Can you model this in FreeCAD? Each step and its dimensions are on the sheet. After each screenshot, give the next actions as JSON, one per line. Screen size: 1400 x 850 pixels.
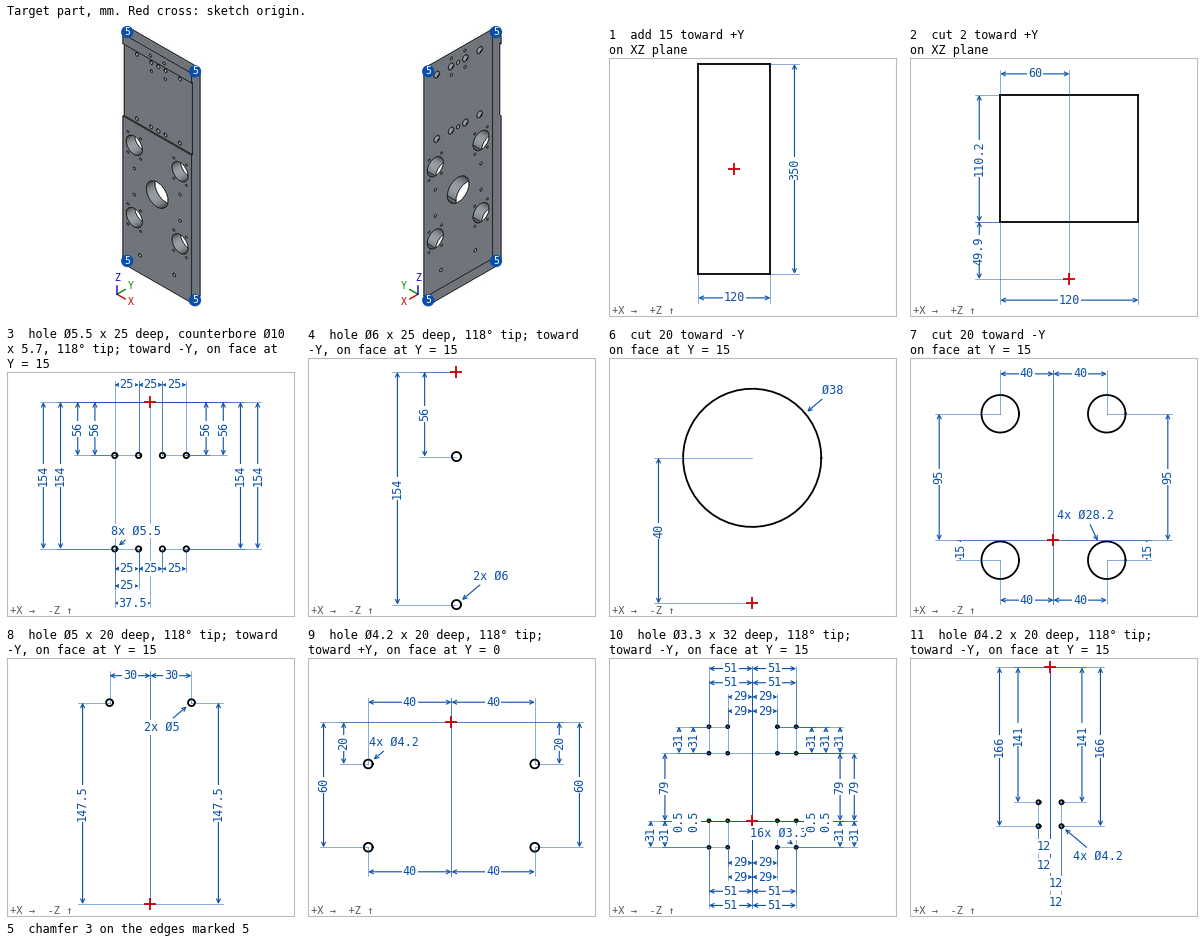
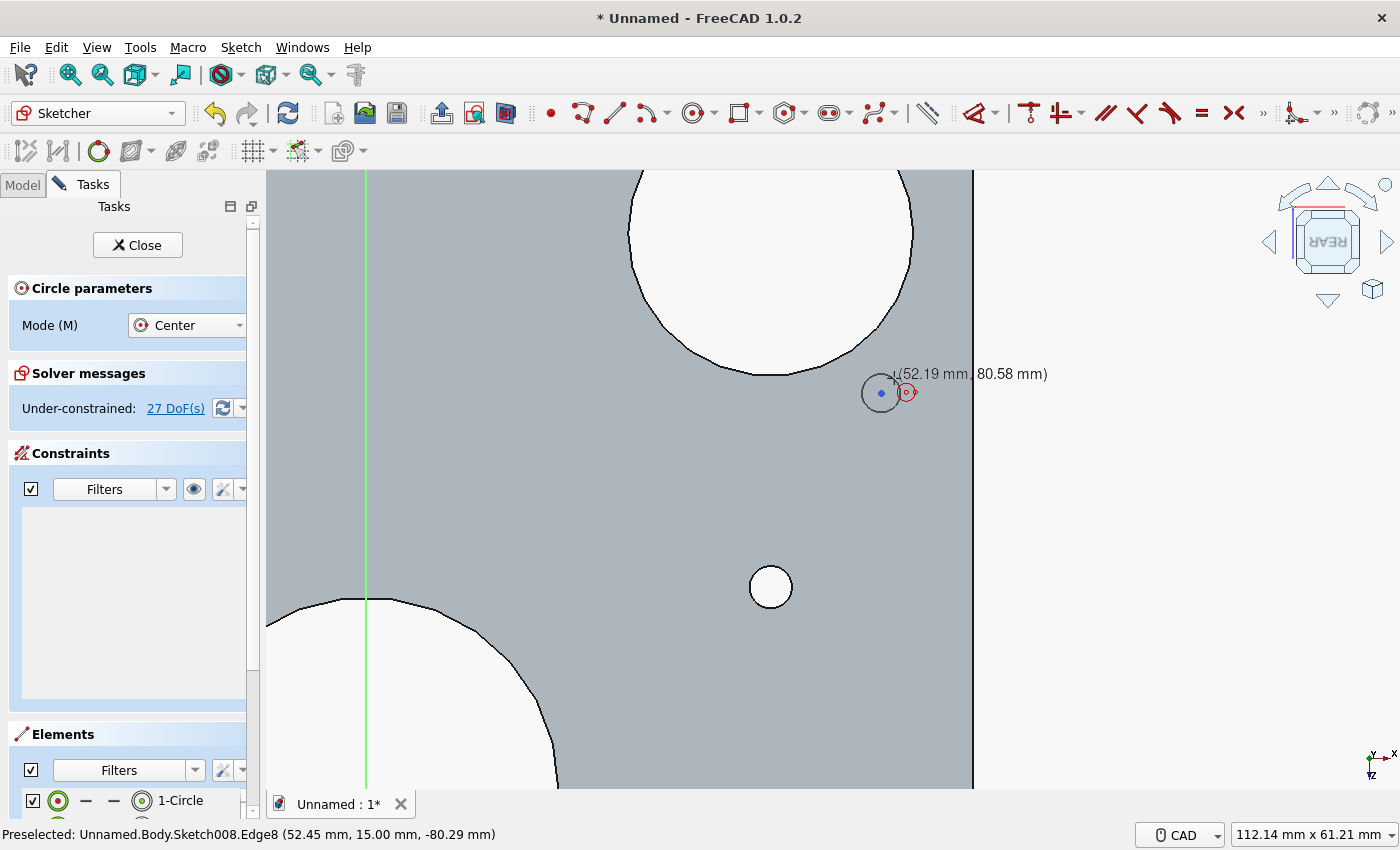
{"action": "scroll", "coordinate": [660, 390], "scroll_direction": "up", "scroll_amount": 2}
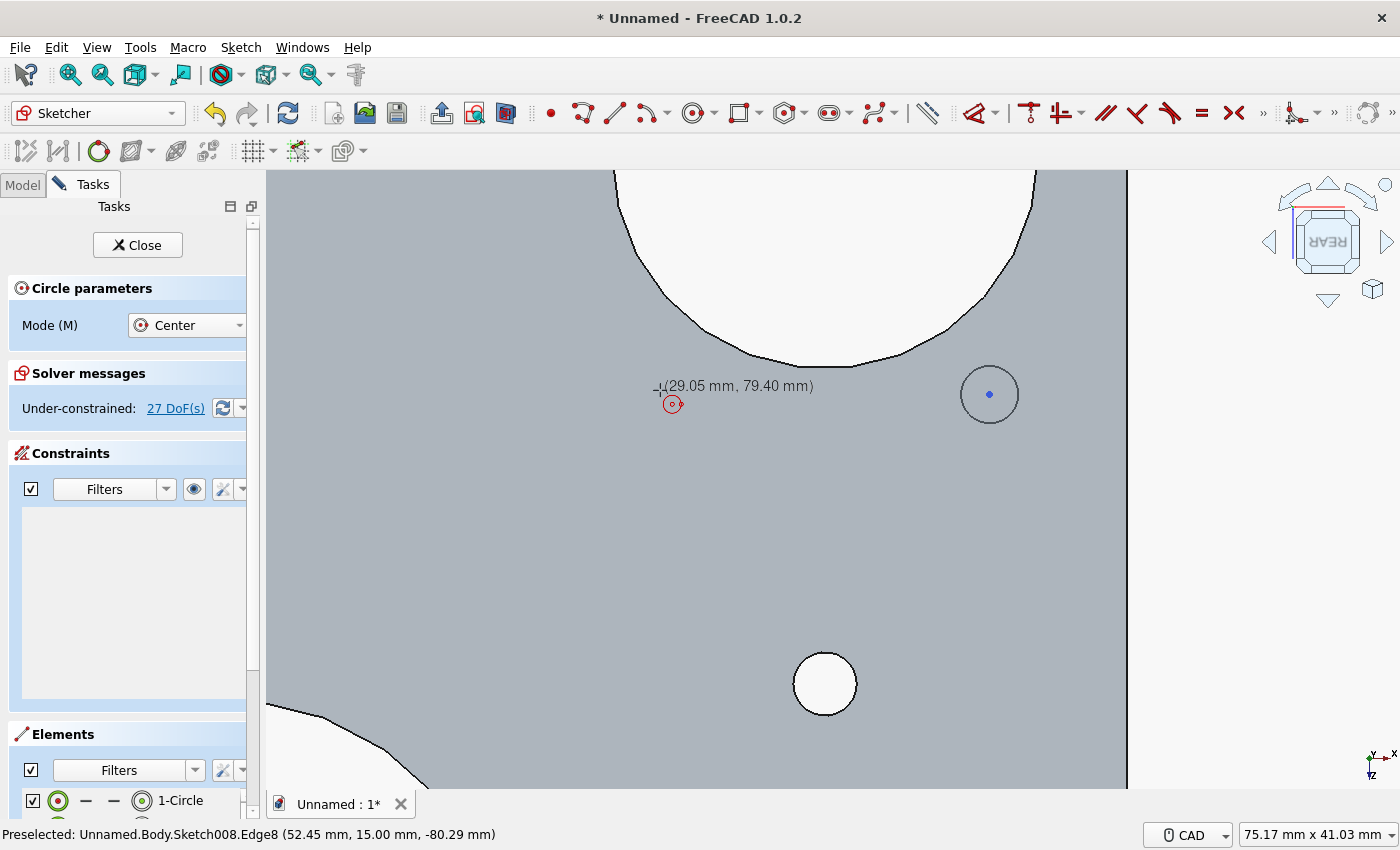
{"action": "scroll", "coordinate": [872, 379], "scroll_direction": "down", "scroll_amount": 9}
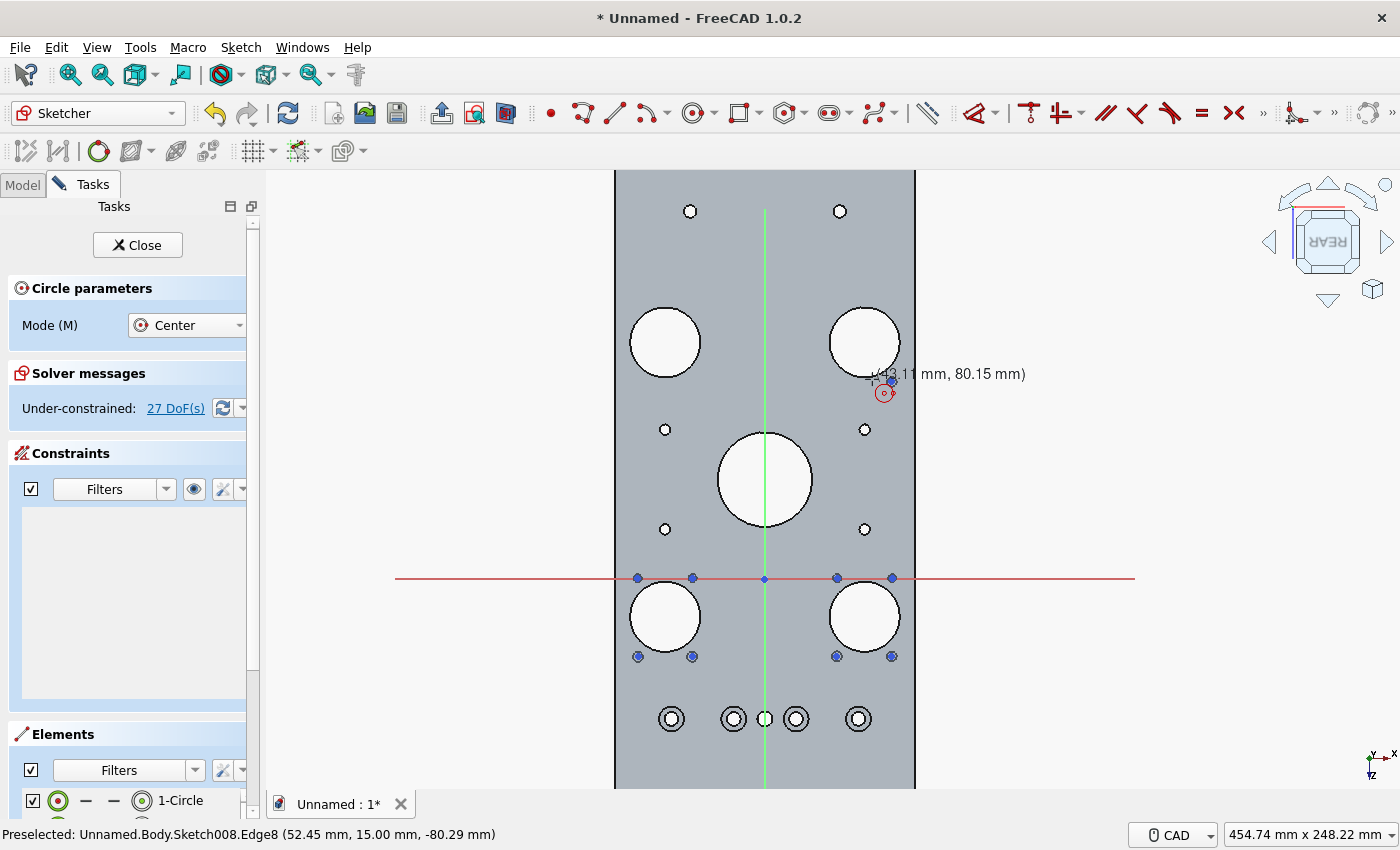
{"action": "left_click", "coordinate": [837, 381]}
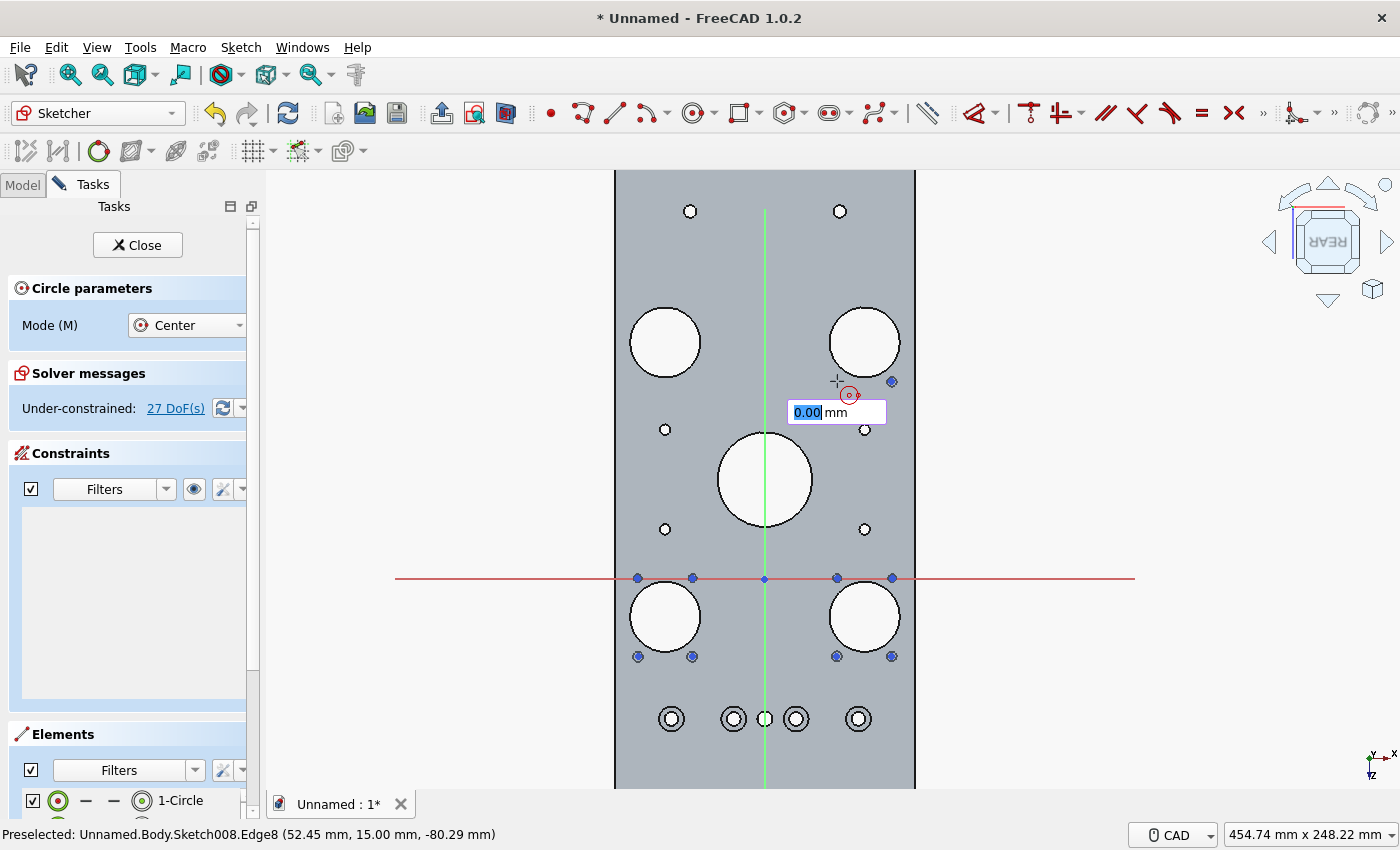
{"action": "scroll", "coordinate": [840, 378], "scroll_direction": "up", "scroll_amount": 7}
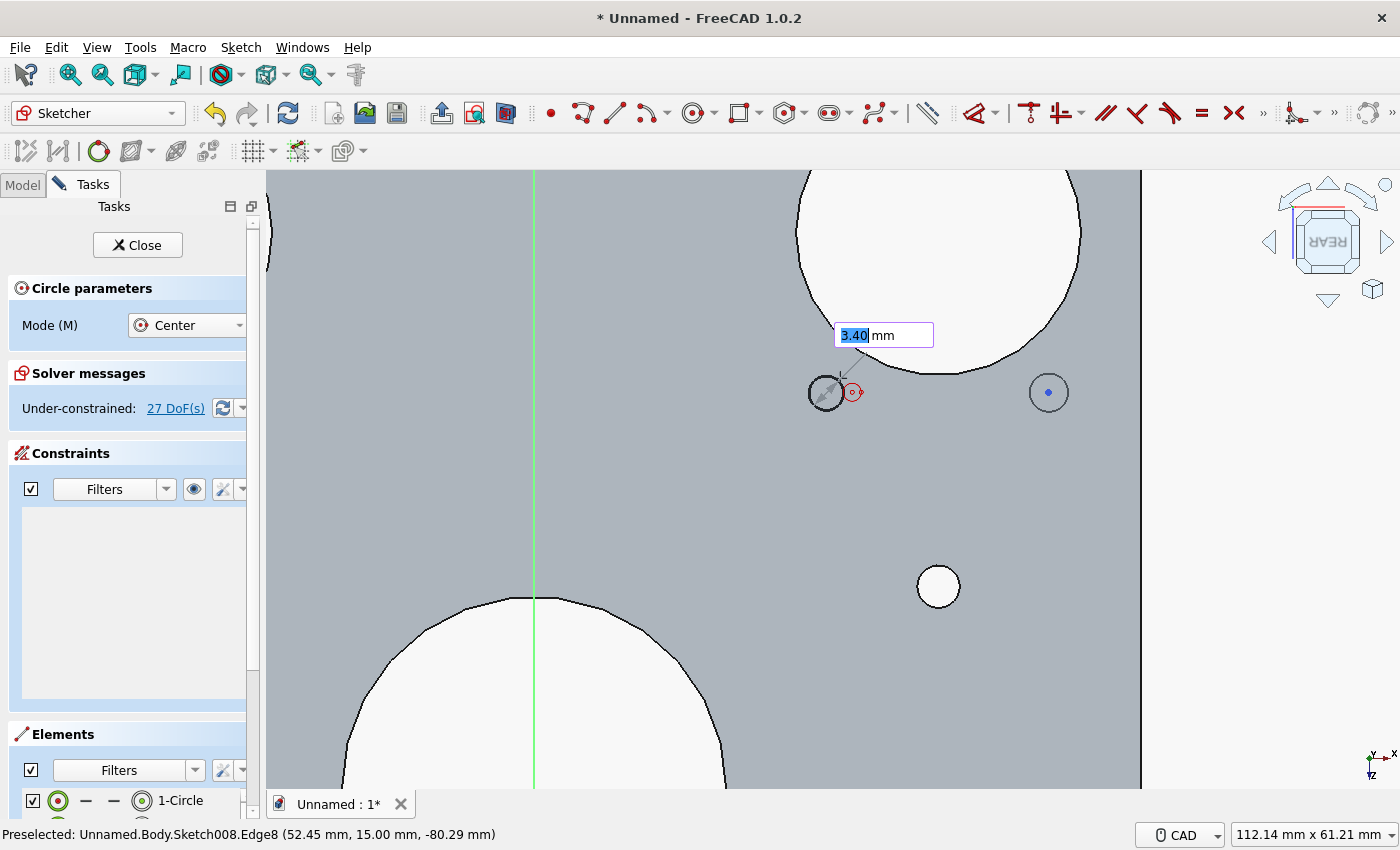
{"action": "left_click", "coordinate": [839, 378]}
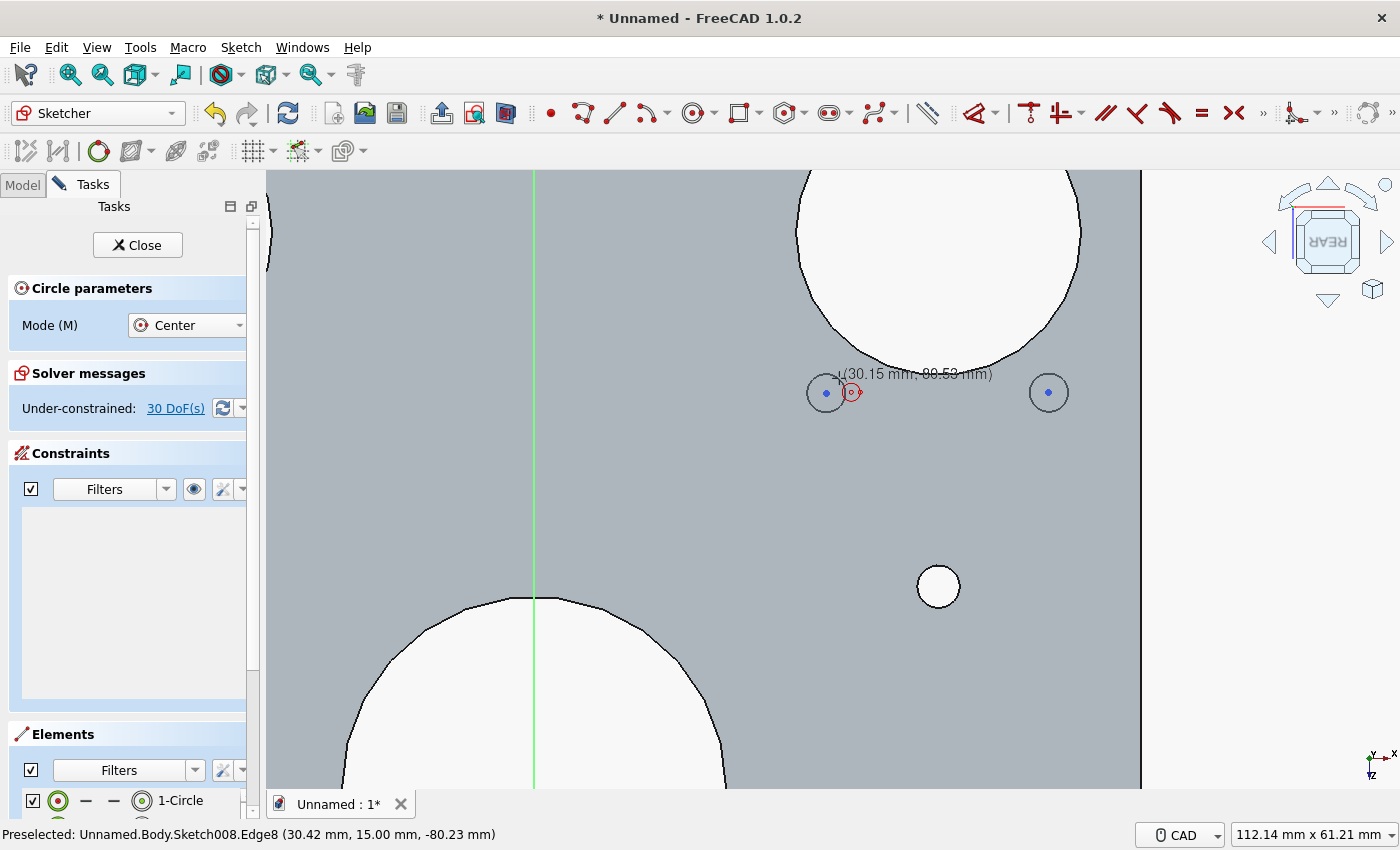
{"action": "scroll", "coordinate": [840, 378], "scroll_direction": "down", "scroll_amount": 7}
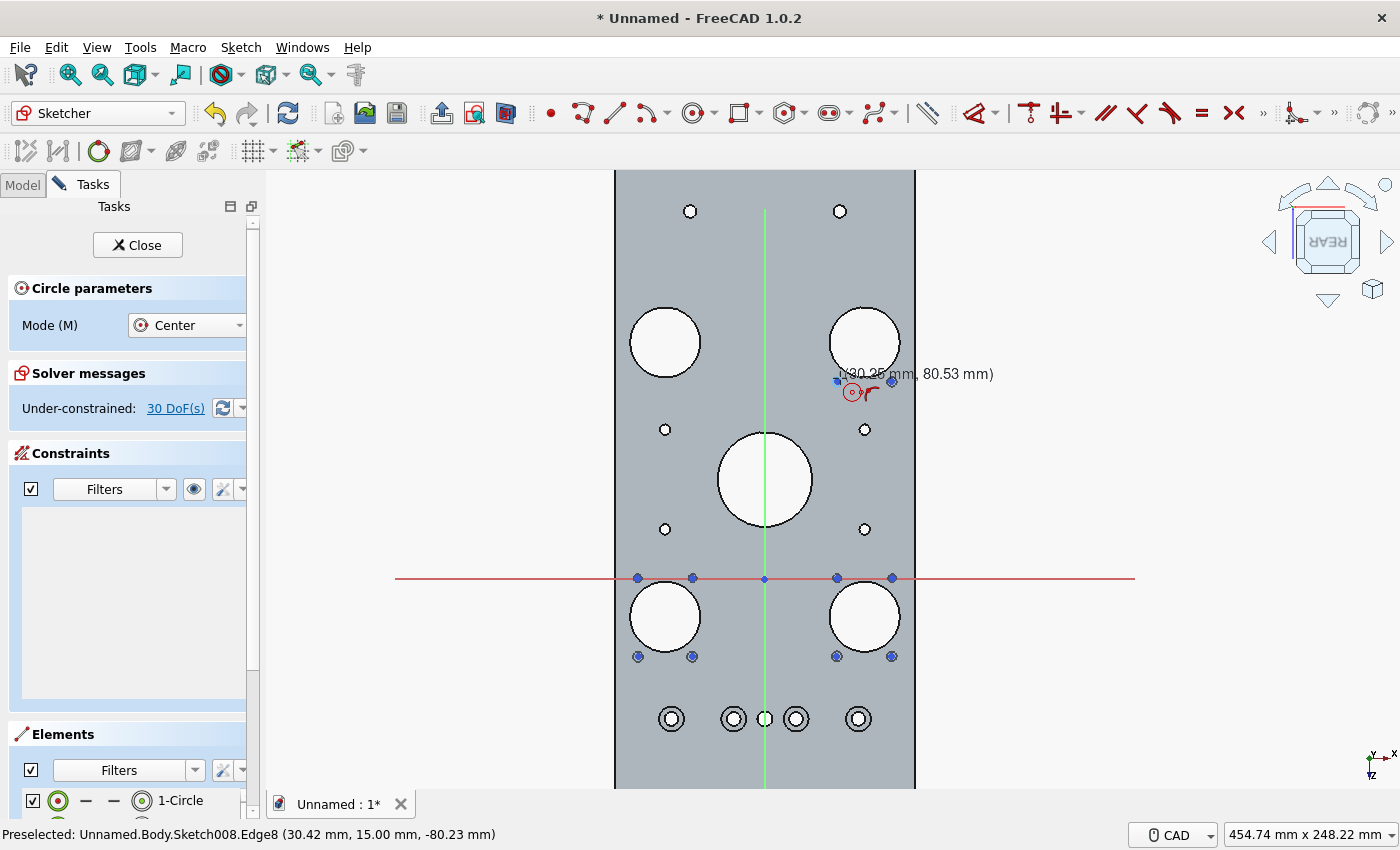
{"action": "scroll", "coordinate": [892, 304], "scroll_direction": "up", "scroll_amount": 9}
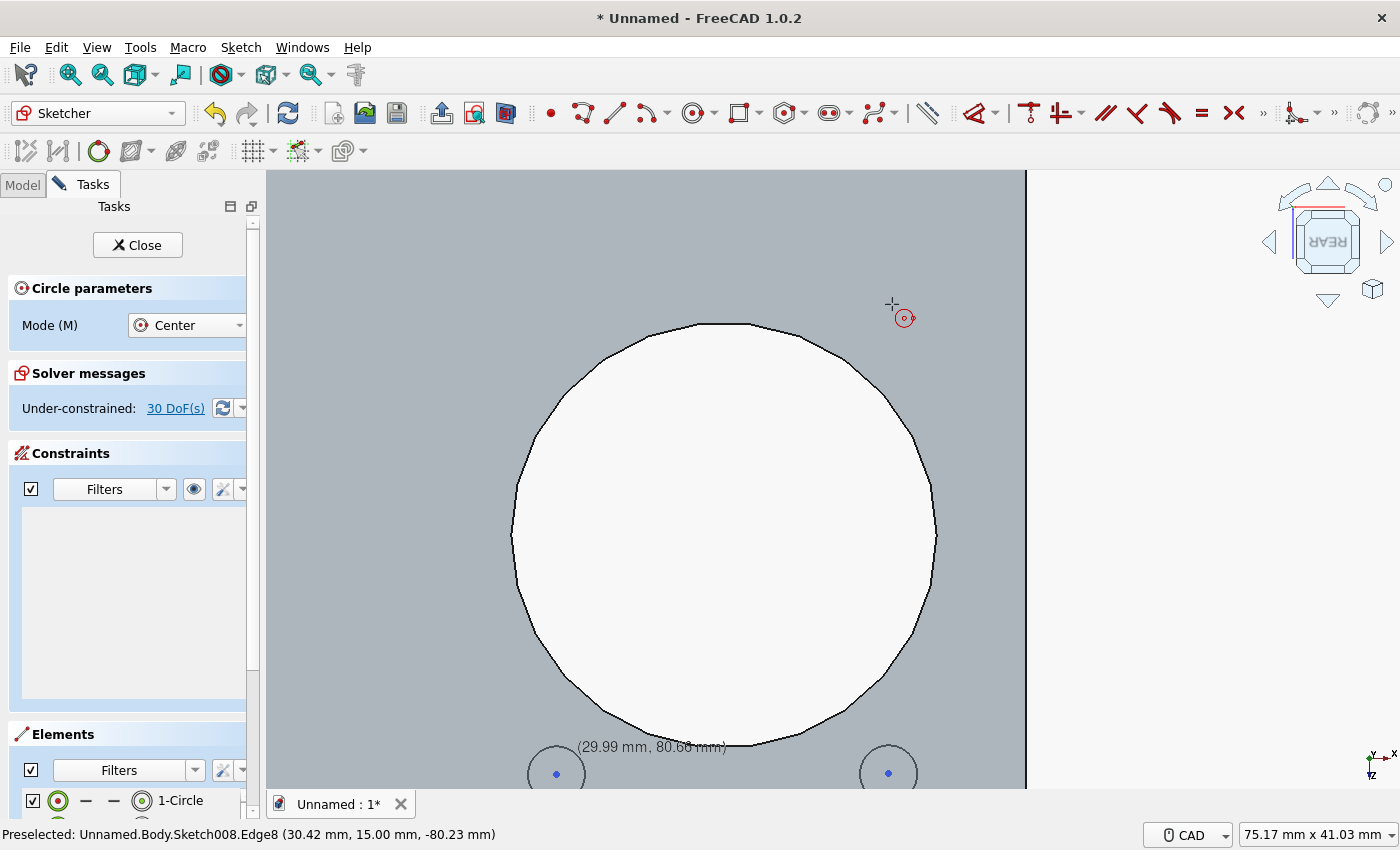
{"action": "scroll", "coordinate": [892, 304], "scroll_direction": "down", "scroll_amount": 9}